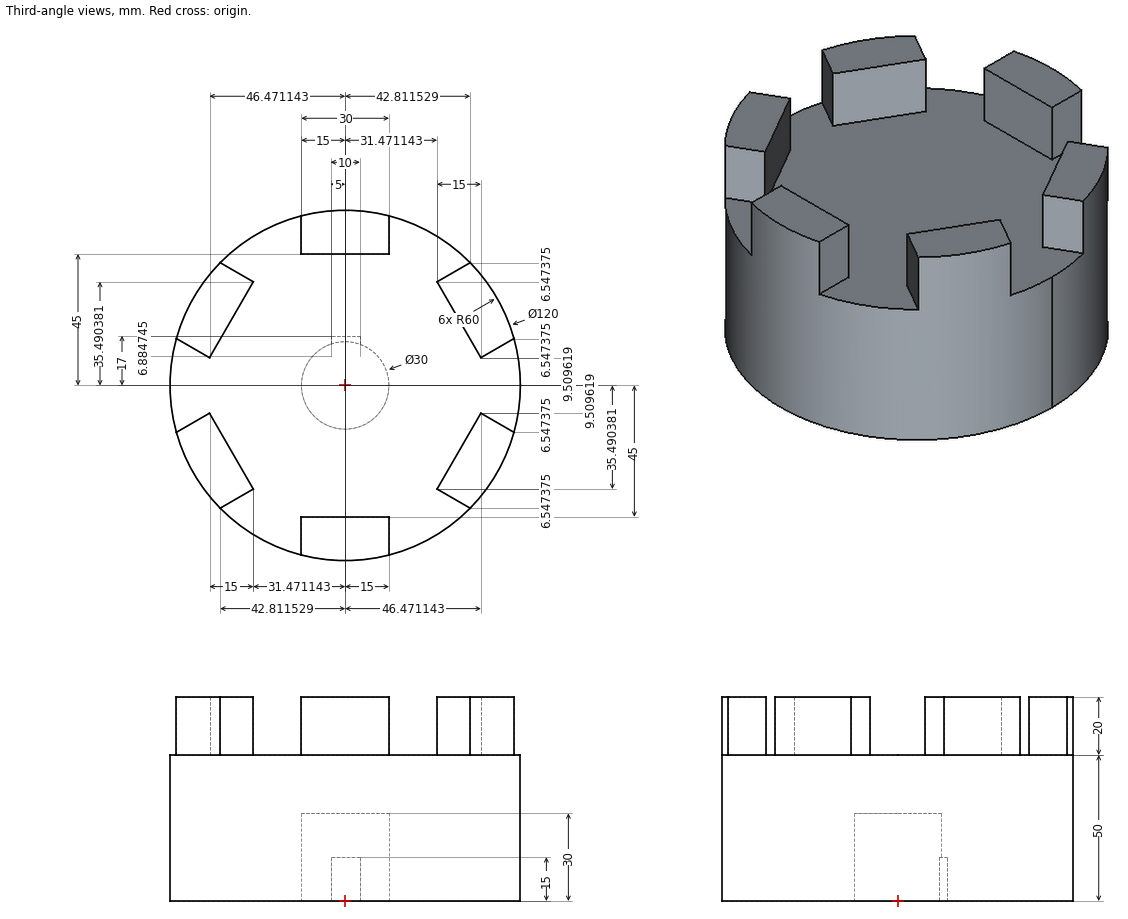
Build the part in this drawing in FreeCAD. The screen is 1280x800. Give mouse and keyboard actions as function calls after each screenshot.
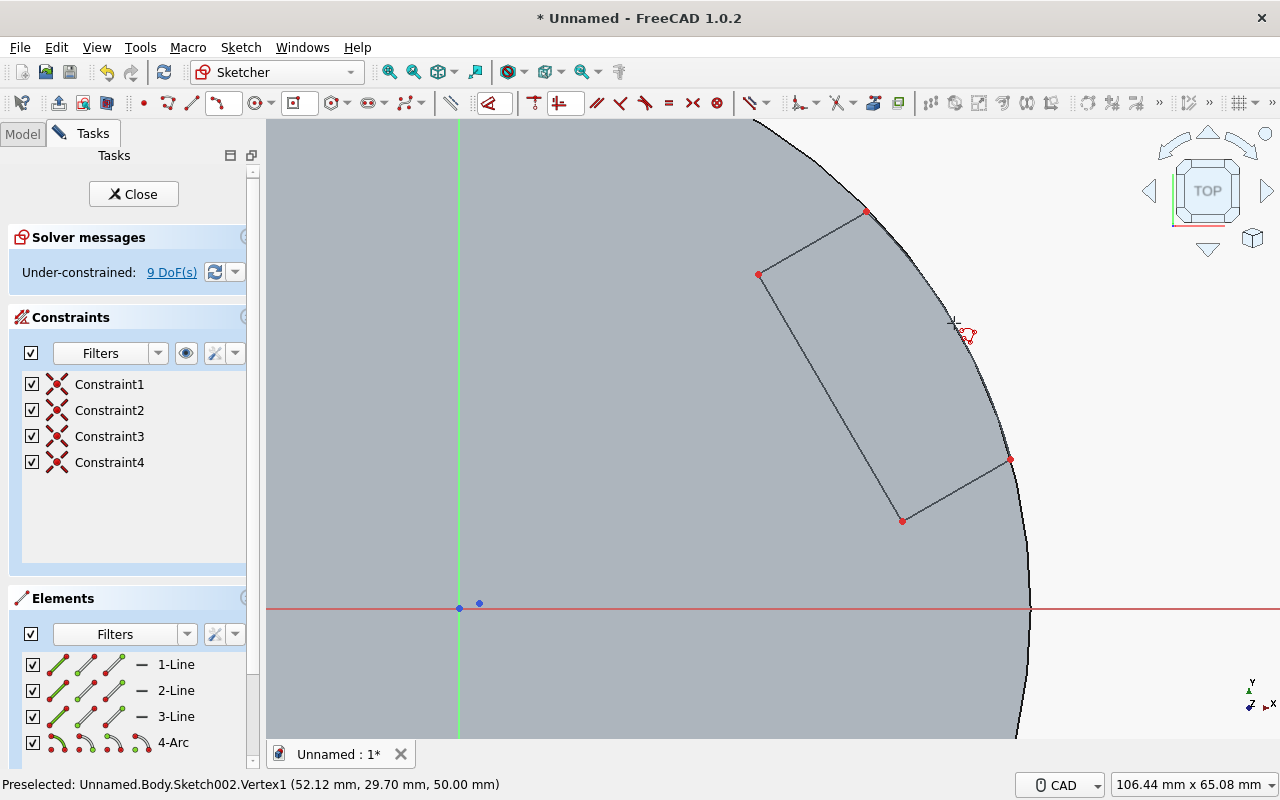
scroll(847, 324, down, 5)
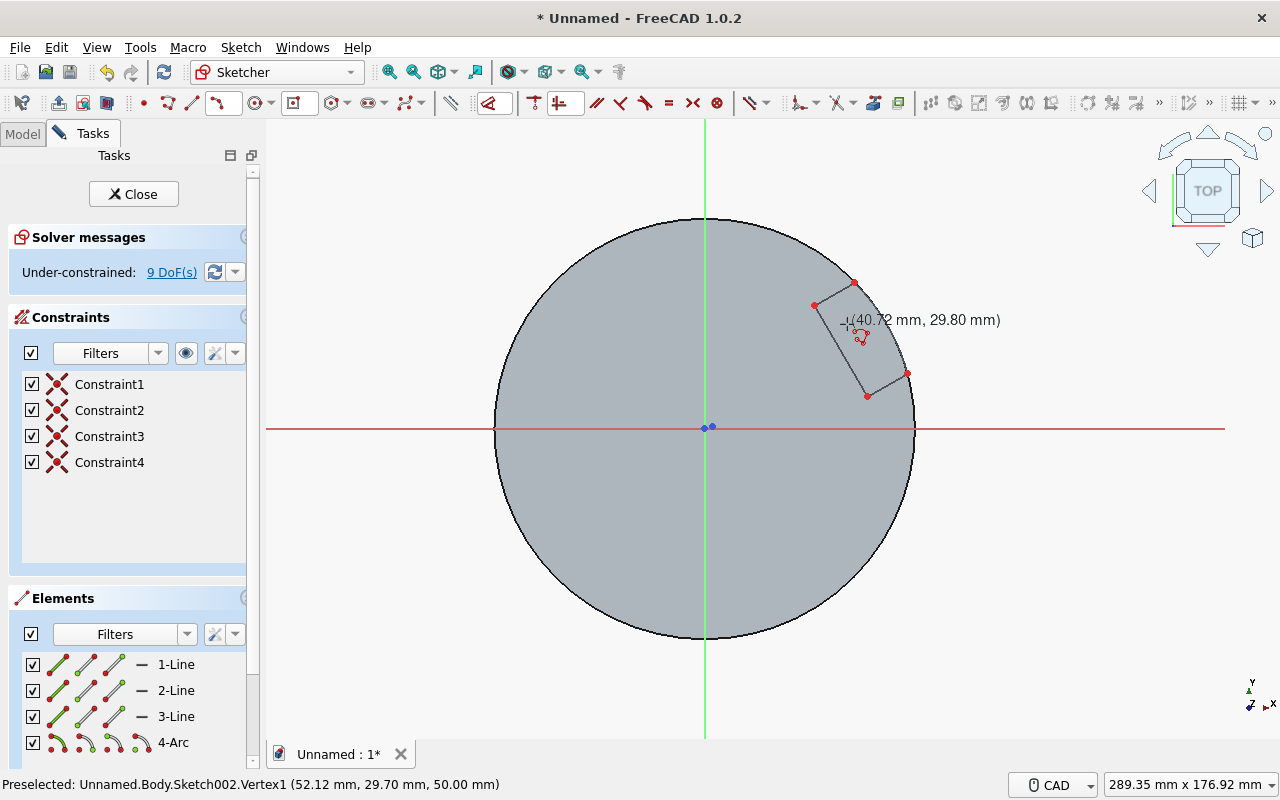
click(652, 225)
click(652, 271)
click(757, 271)
click(757, 225)
right_click(757, 225)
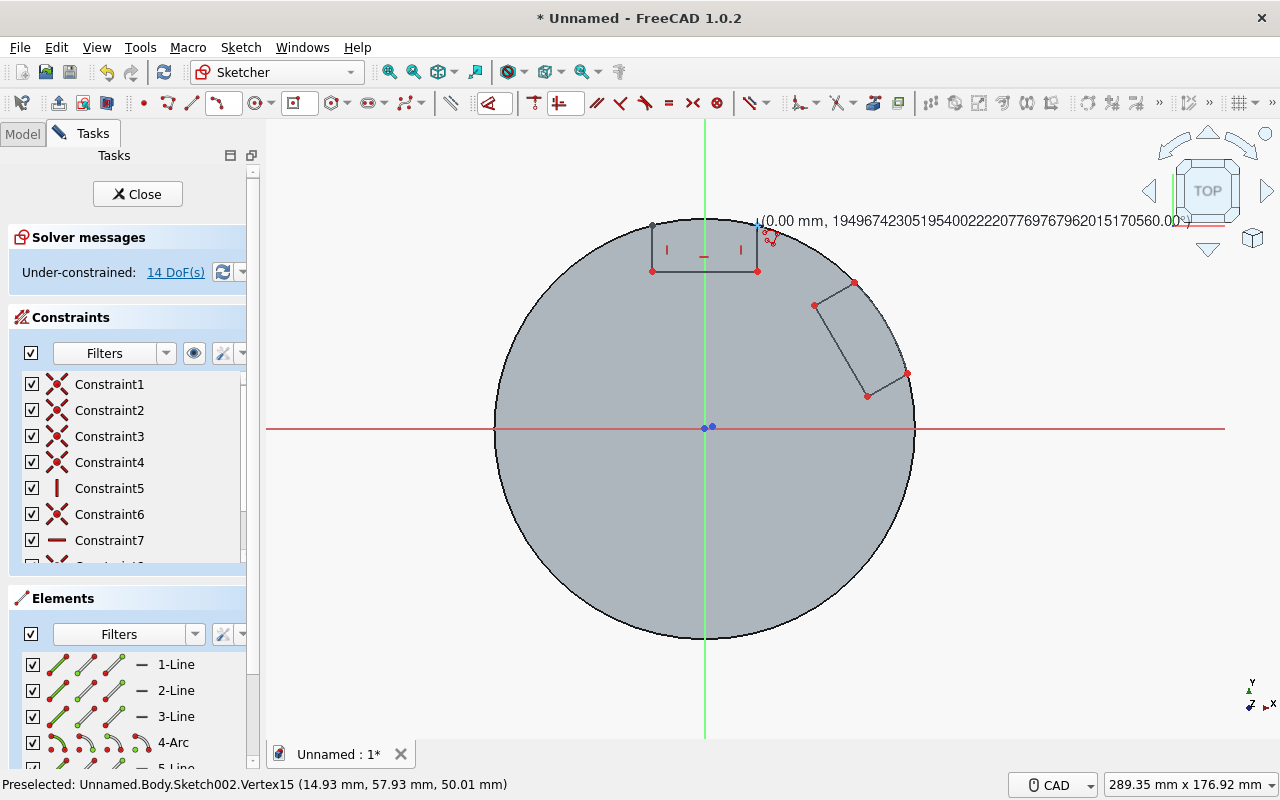
key(g)
key(3)
key(a)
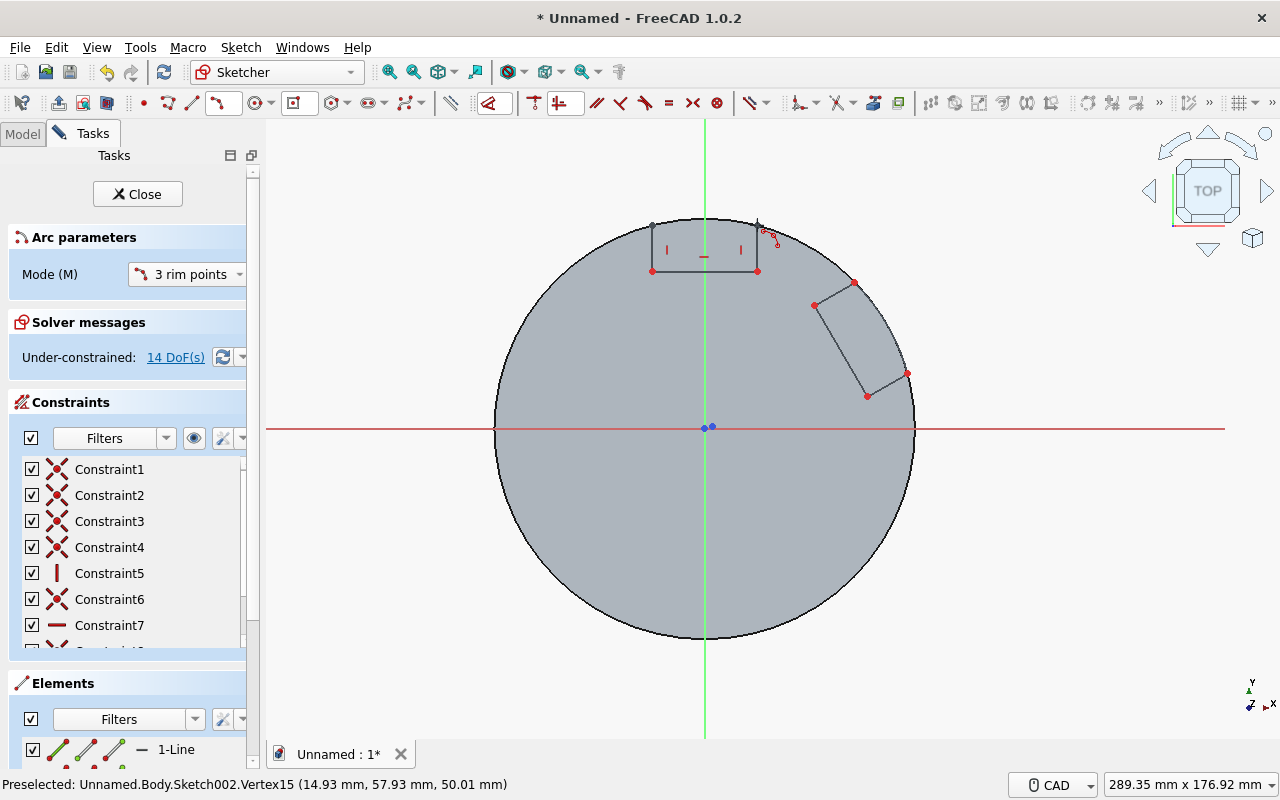
click(757, 226)
click(652, 226)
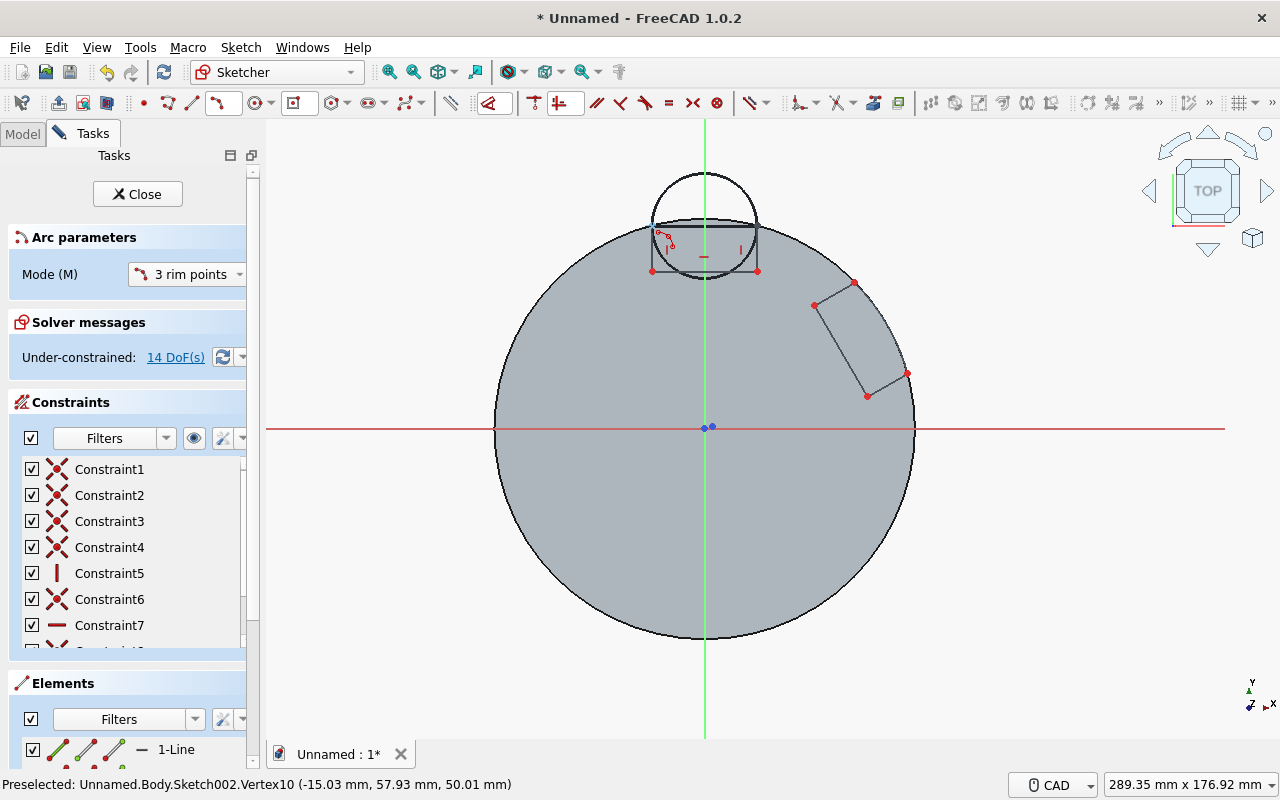
scroll(715, 219, up, 5)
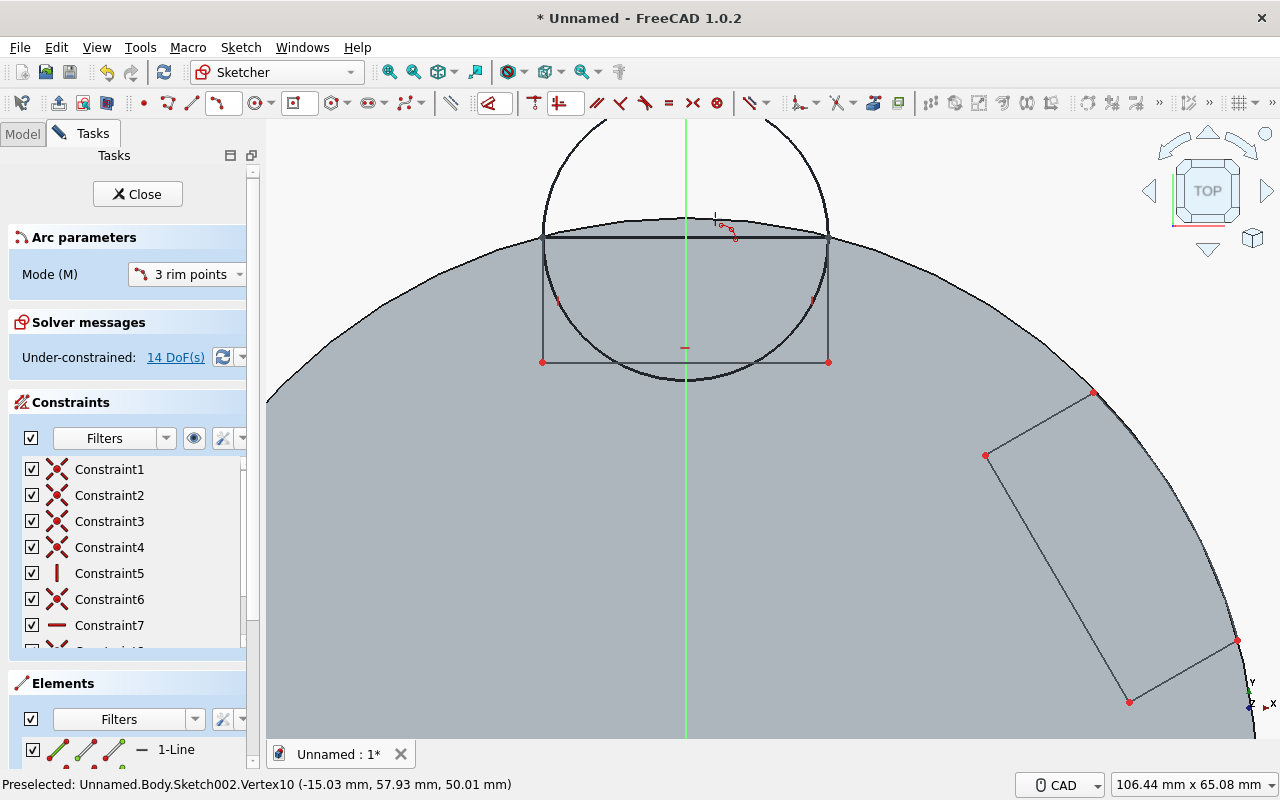
click(715, 219)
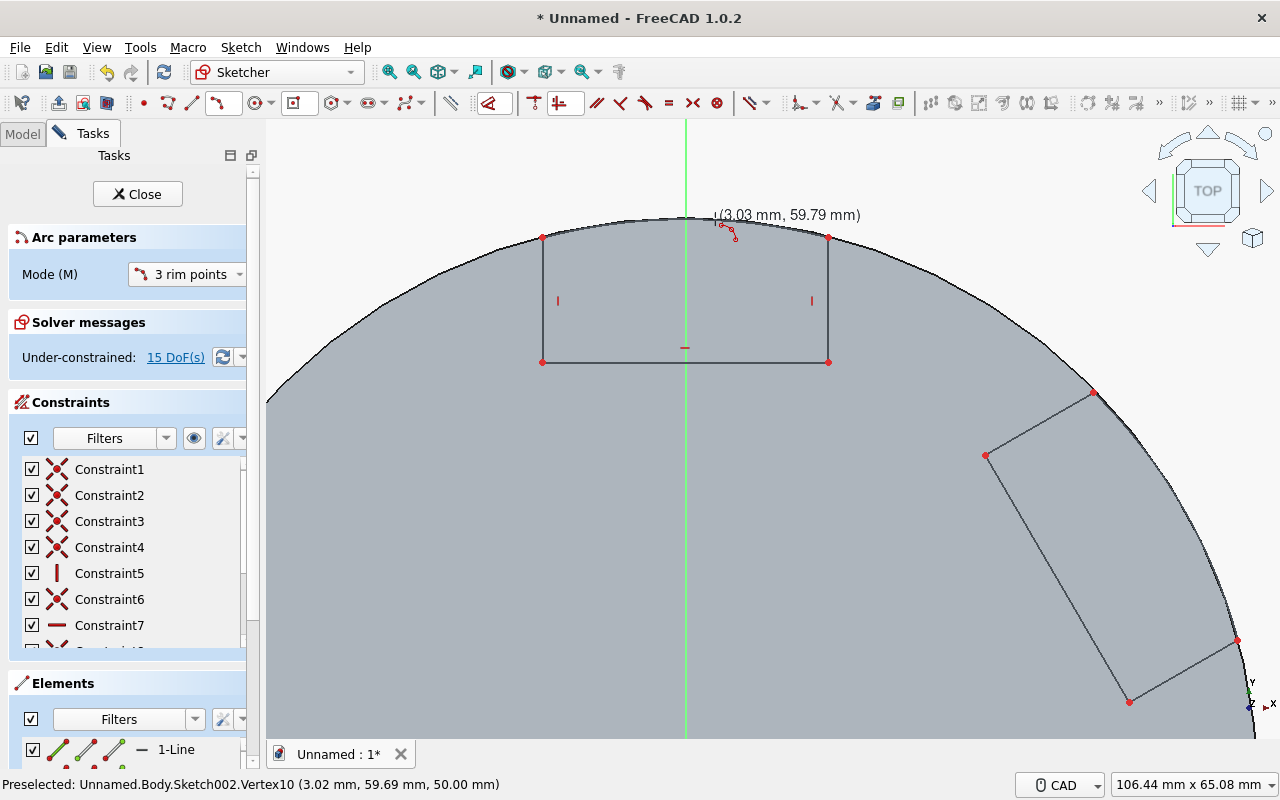
key(g)
key(m)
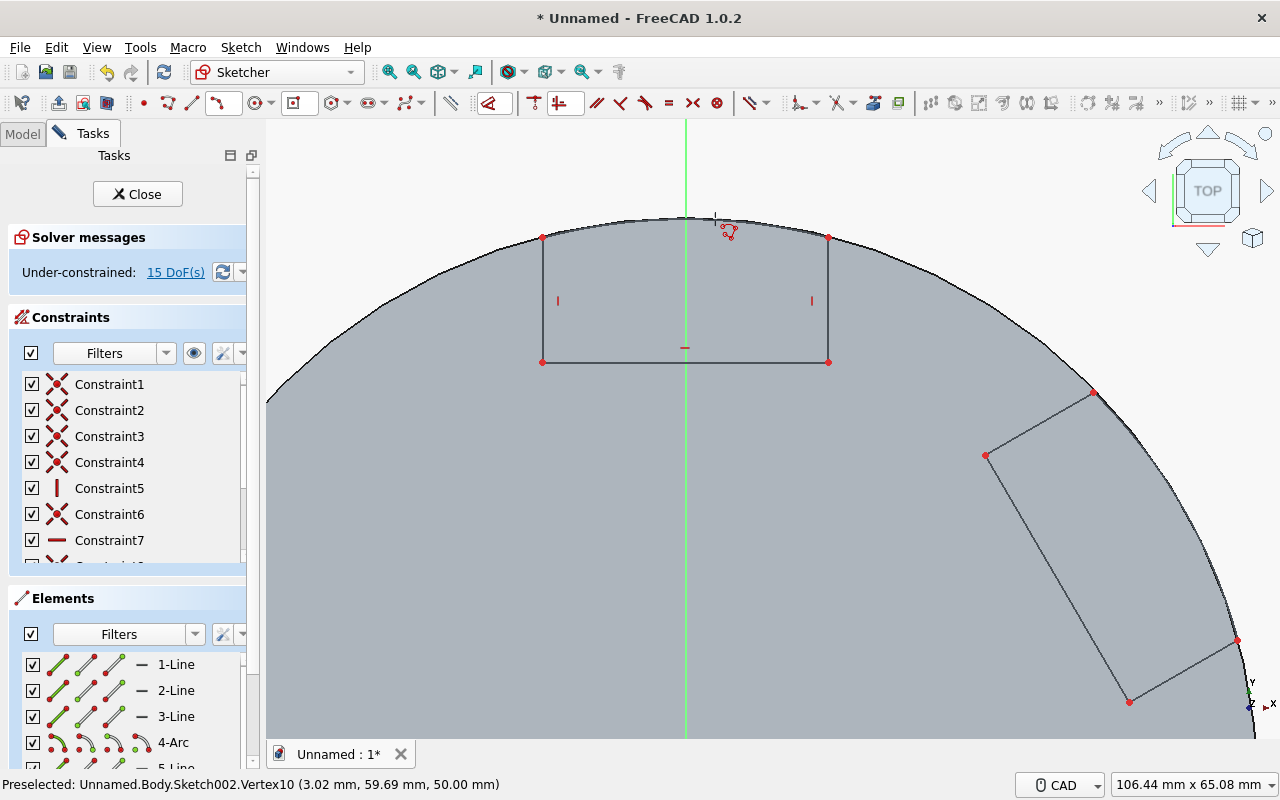
scroll(715, 219, down, 5)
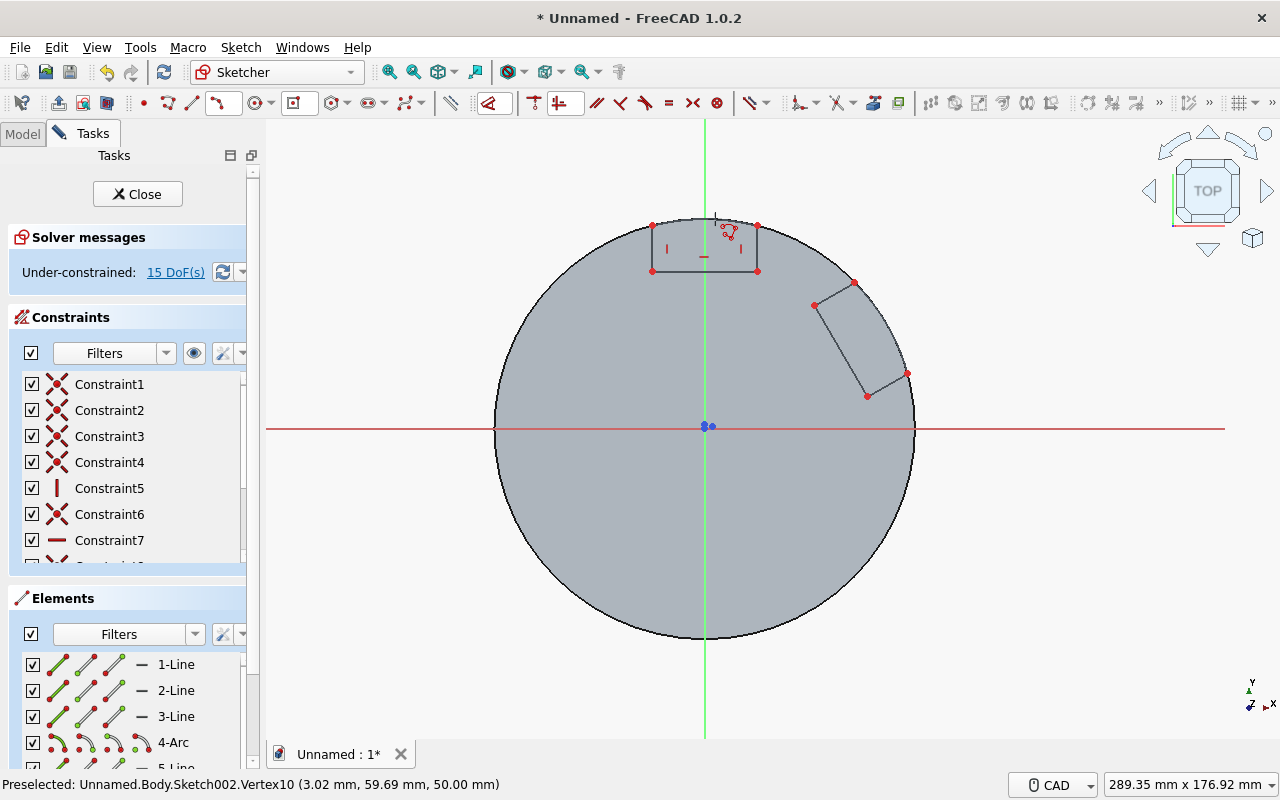
click(907, 485)
click(868, 462)
click(815, 553)
click(855, 576)
right_click(855, 576)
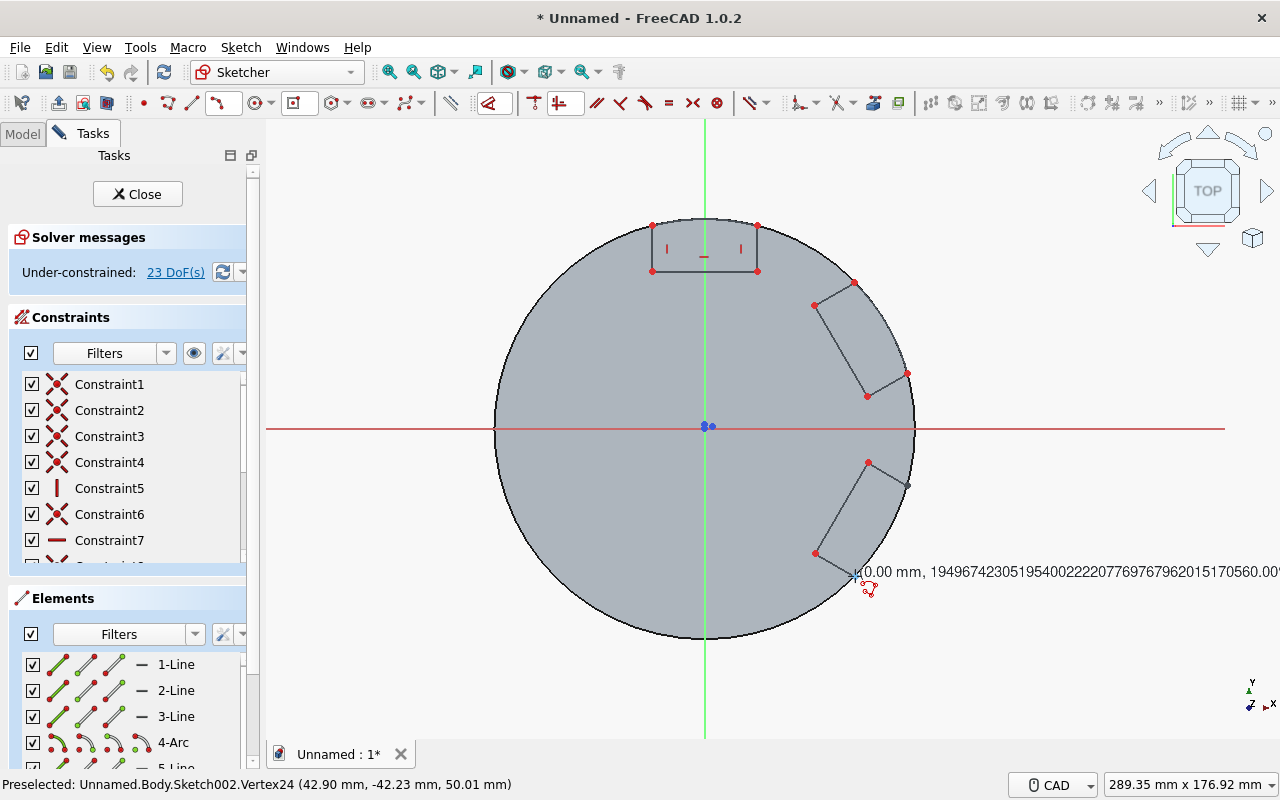
key(g)
key(3)
key(a)